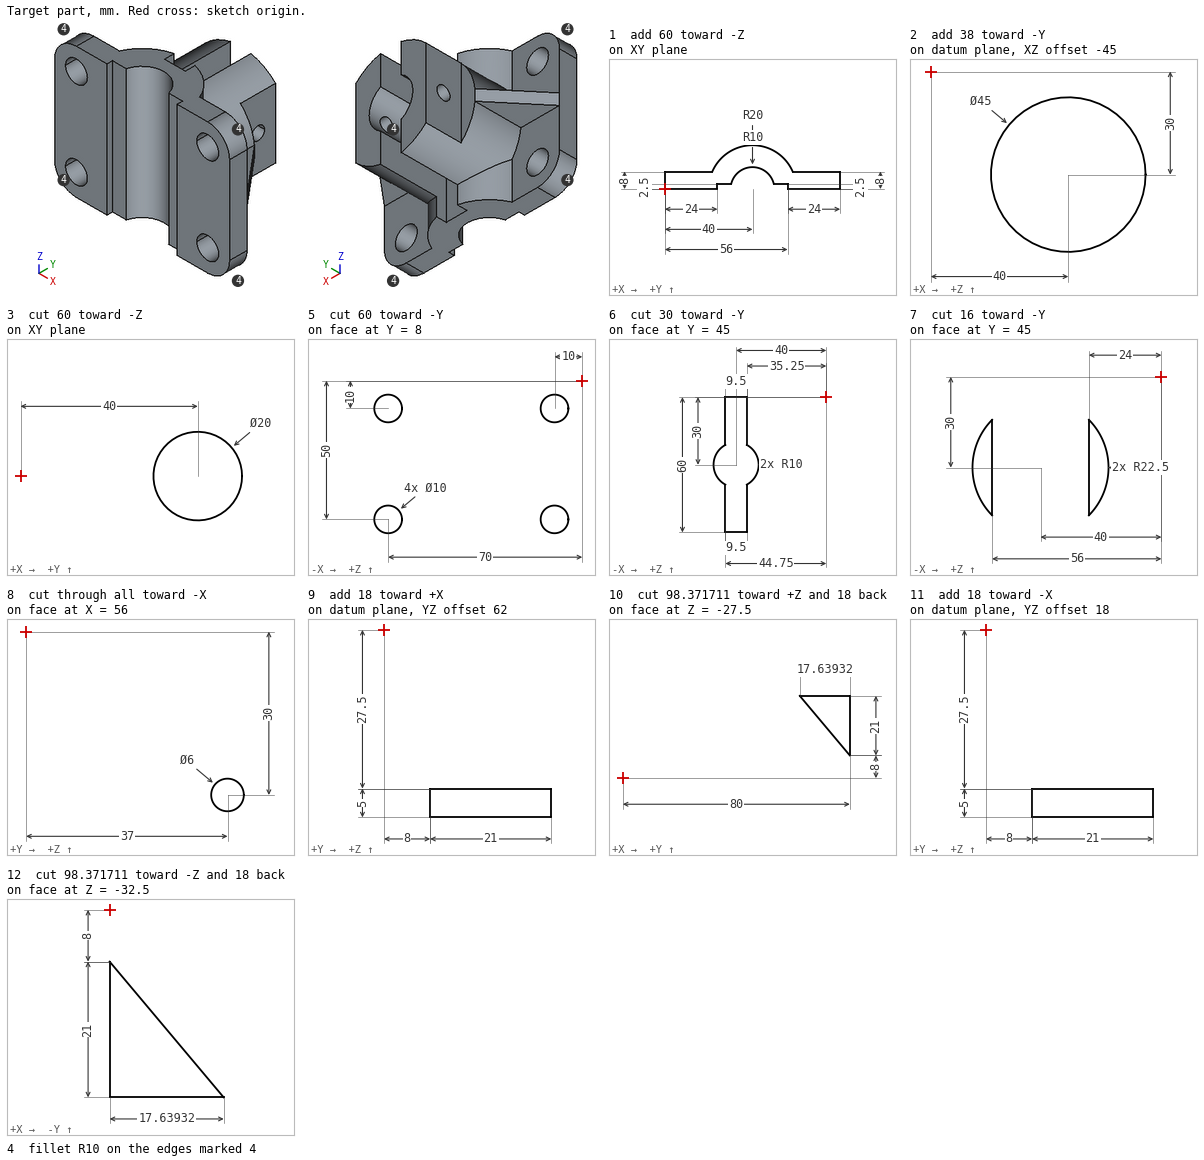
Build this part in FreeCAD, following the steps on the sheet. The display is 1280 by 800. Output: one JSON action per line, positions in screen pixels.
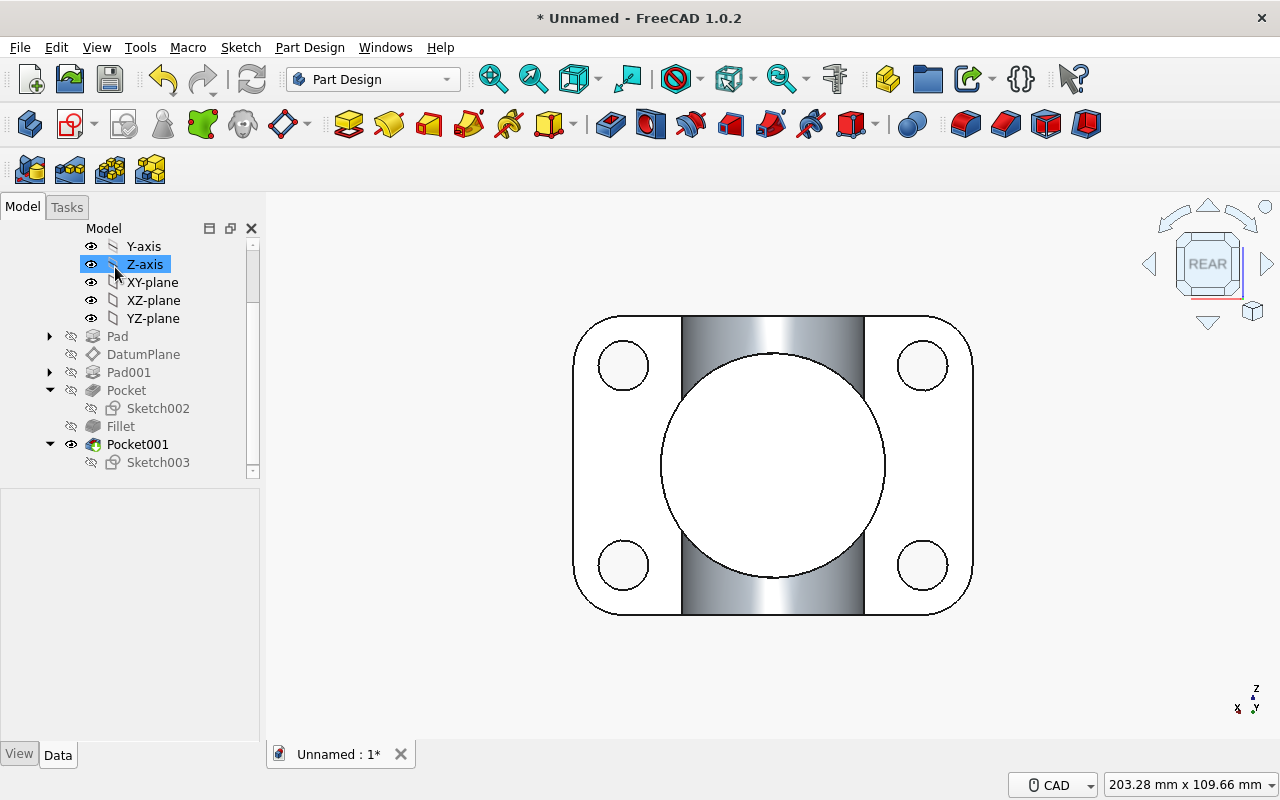
{"action": "left_click", "coordinate": [773, 464]}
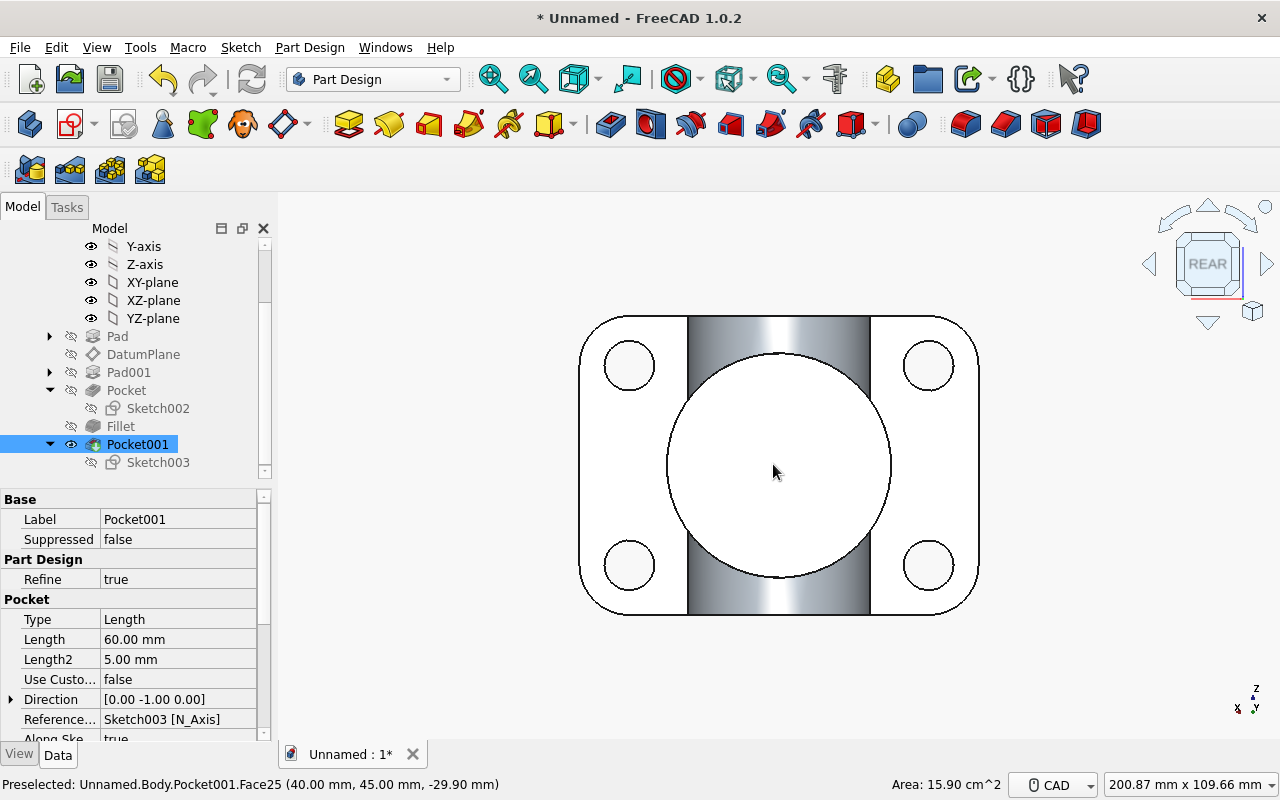
{"action": "left_click", "coordinate": [70, 124]}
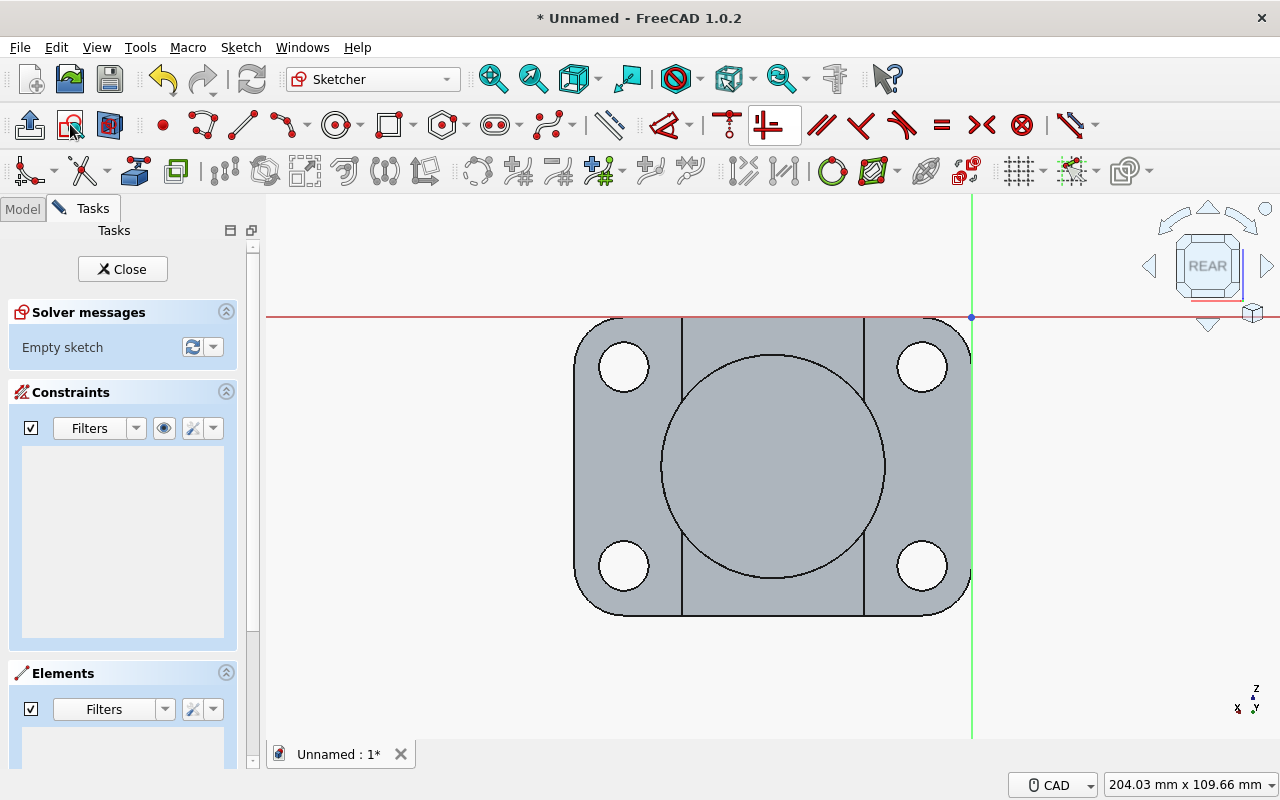
{"action": "left_click", "coordinate": [204, 126]}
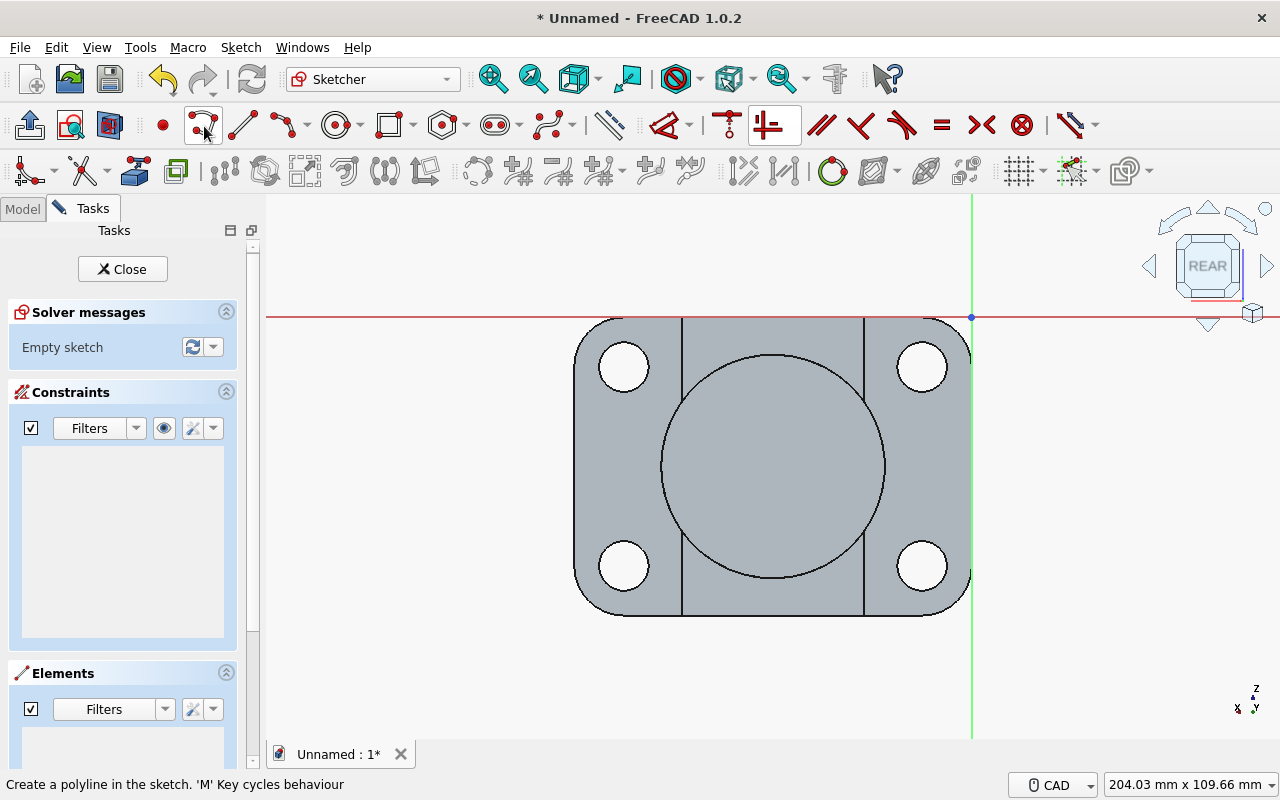
{"action": "left_click", "coordinate": [797, 423]}
{"action": "left_click", "coordinate": [797, 317]}
{"action": "left_click", "coordinate": [749, 326]}
{"action": "left_click", "coordinate": [749, 423]}
{"action": "right_click", "coordinate": [749, 423]}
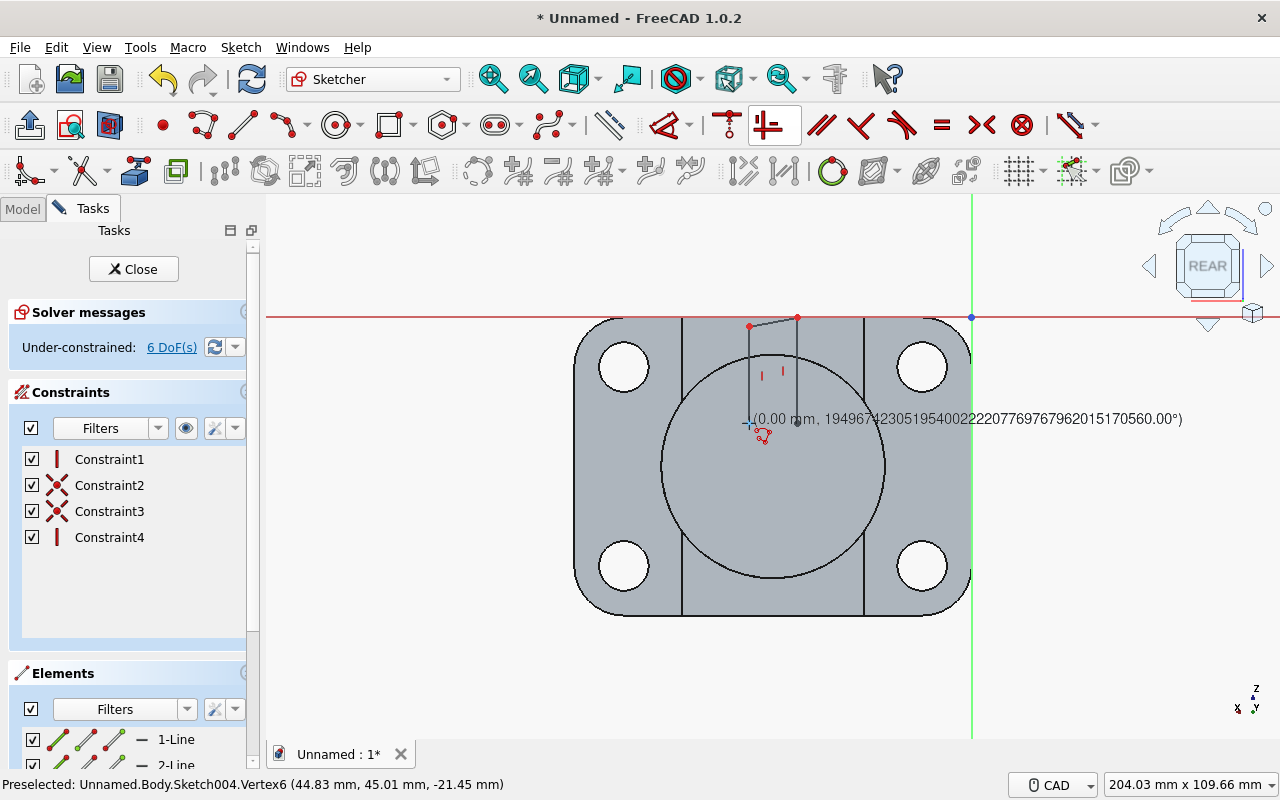
{"action": "left_click", "coordinate": [749, 510]}
{"action": "left_click", "coordinate": [749, 616]}
{"action": "left_click", "coordinate": [797, 616]}
{"action": "left_click", "coordinate": [797, 510]}
{"action": "right_click", "coordinate": [797, 510]}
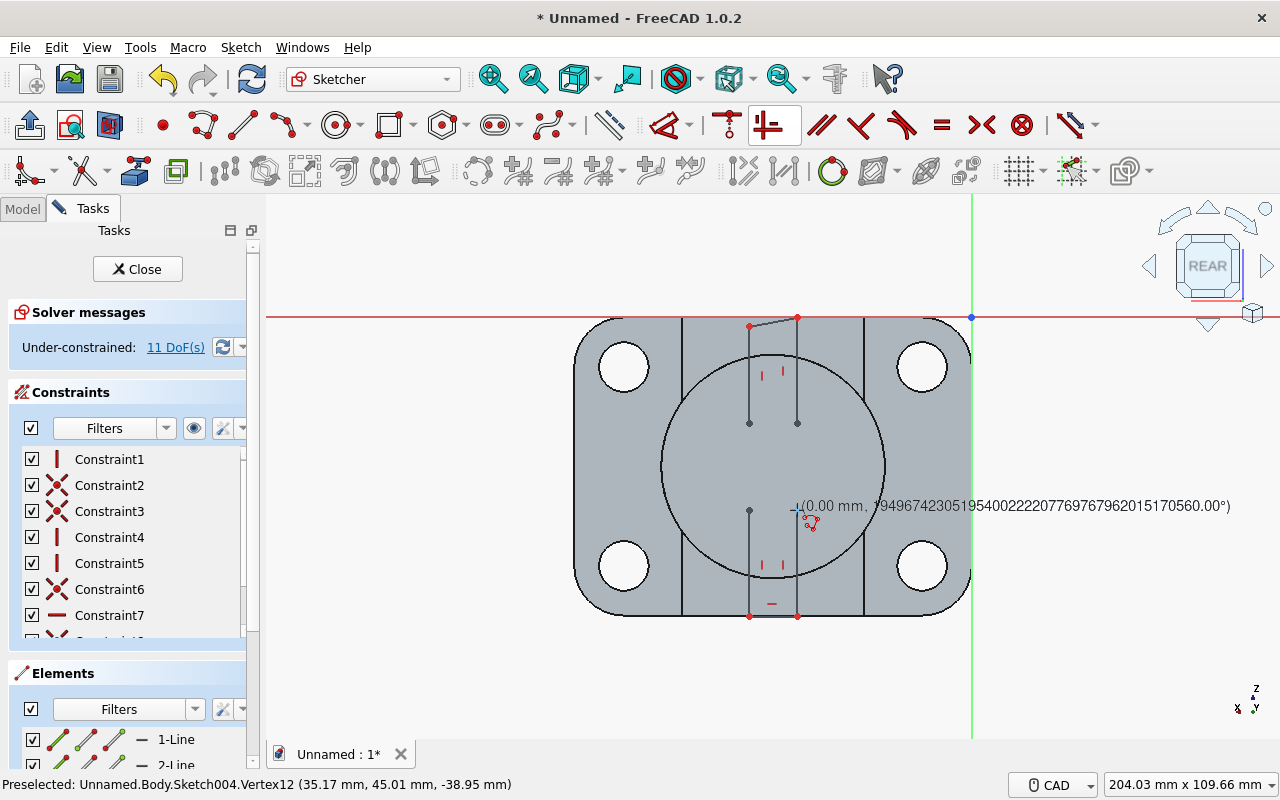
{"action": "left_click", "coordinate": [284, 126]}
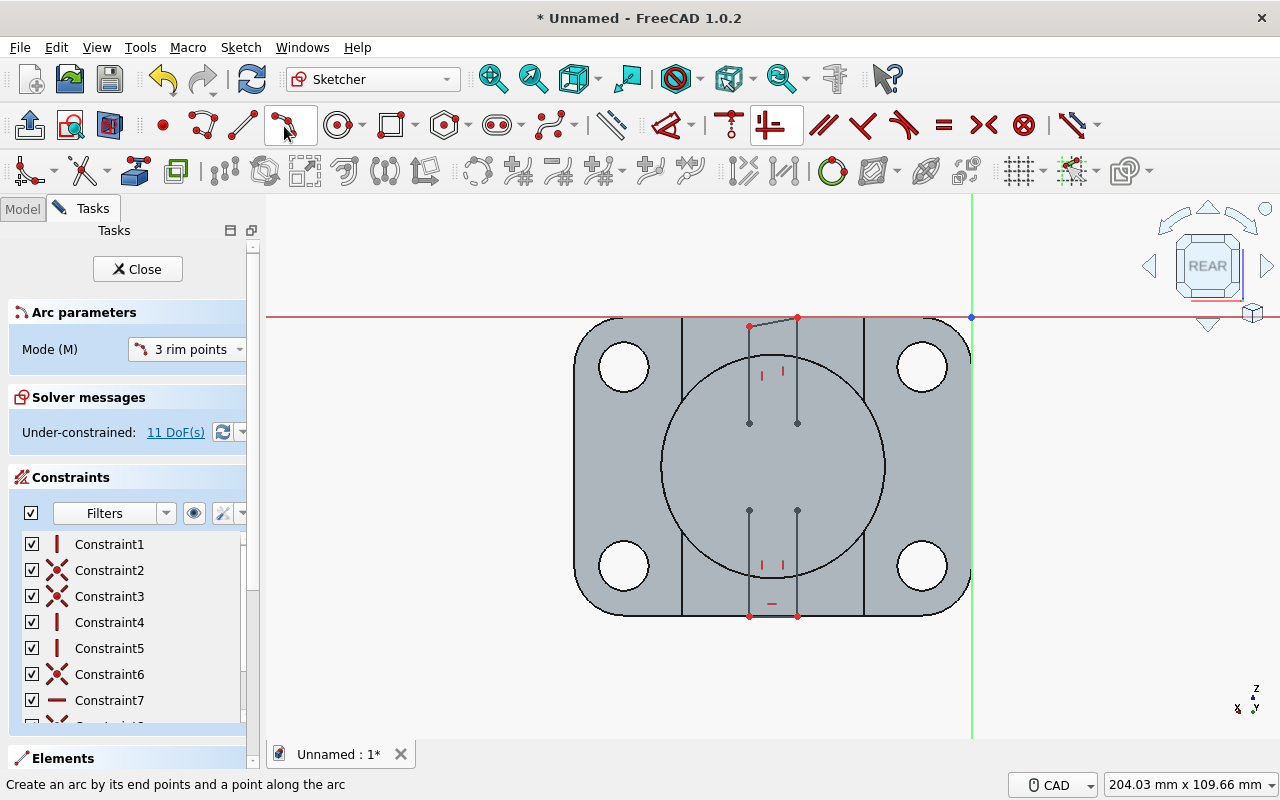
{"action": "left_click", "coordinate": [749, 424]}
{"action": "left_click", "coordinate": [749, 511]}
{"action": "left_click", "coordinate": [723, 467]}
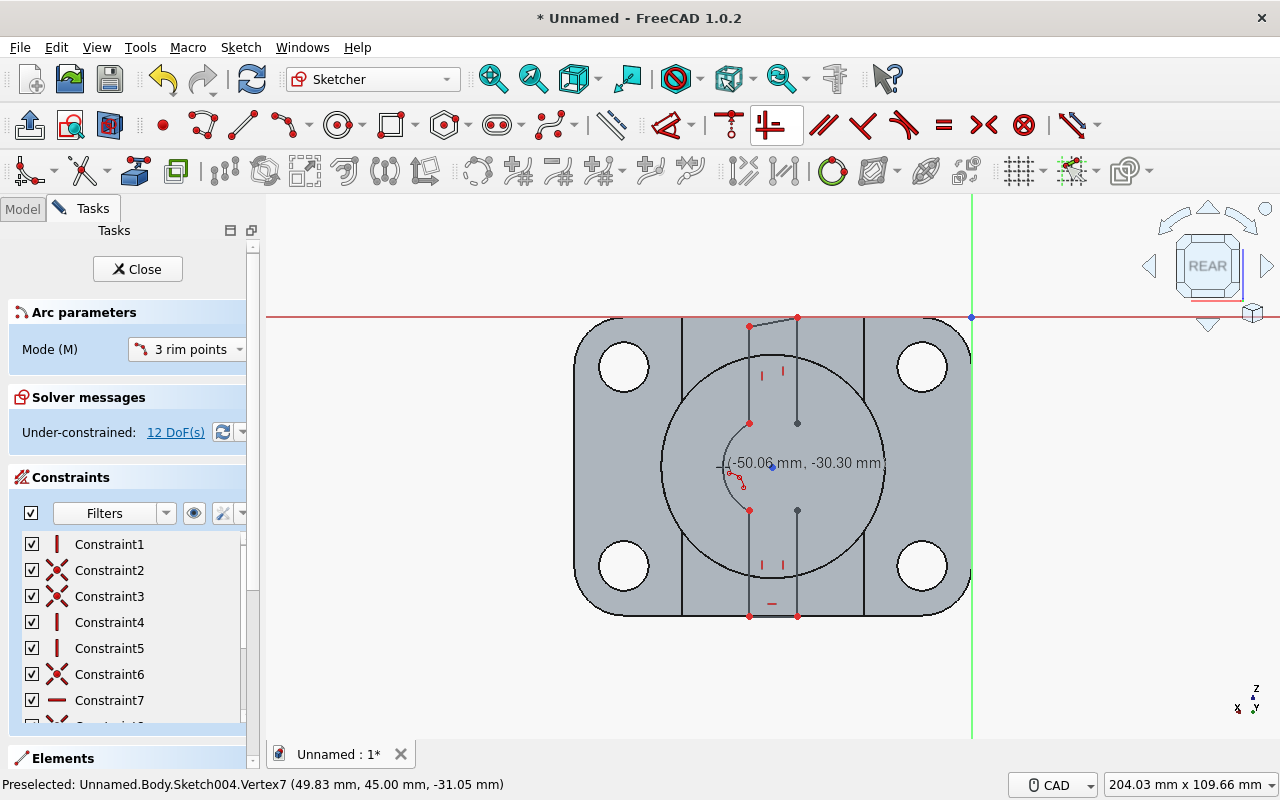
{"action": "left_click", "coordinate": [797, 511]}
{"action": "left_click", "coordinate": [797, 424]}
{"action": "left_click", "coordinate": [823, 467]}
{"action": "key", "text": "Escape"}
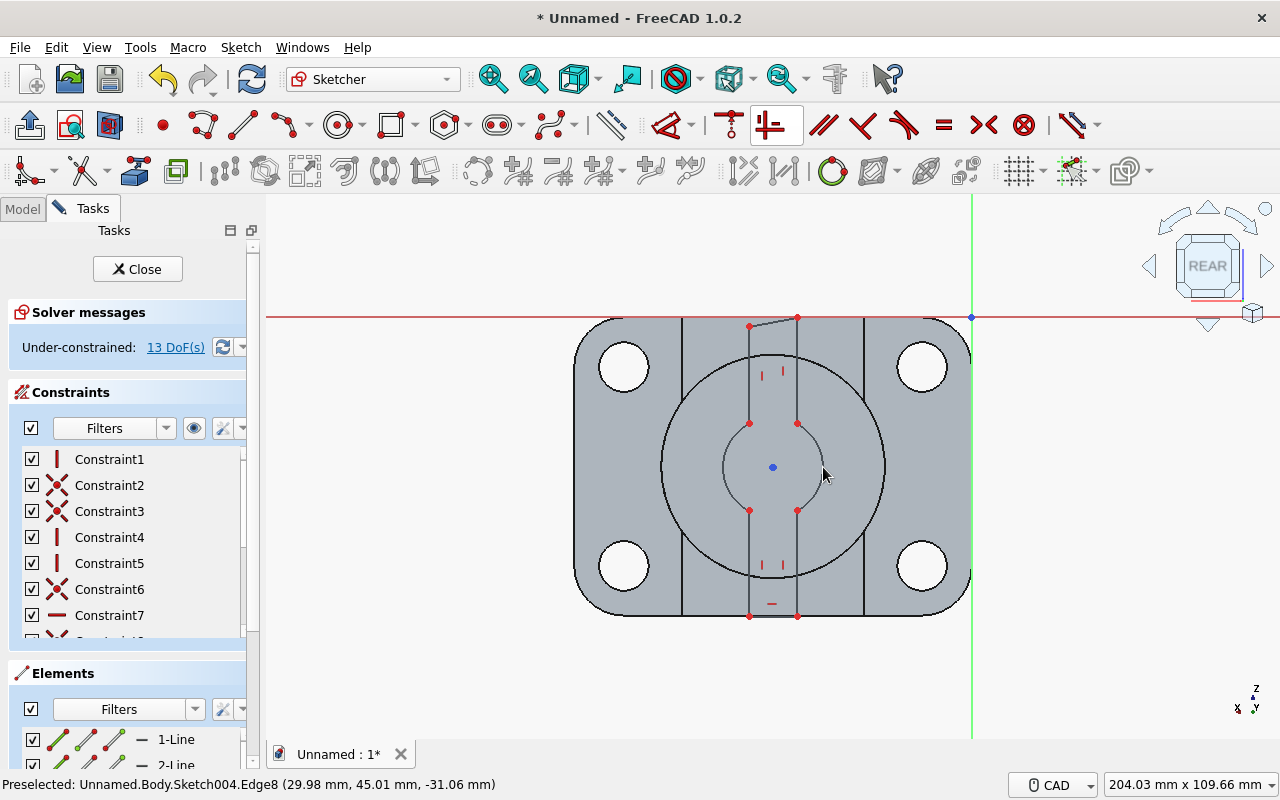
{"action": "left_click", "coordinate": [783, 321]}